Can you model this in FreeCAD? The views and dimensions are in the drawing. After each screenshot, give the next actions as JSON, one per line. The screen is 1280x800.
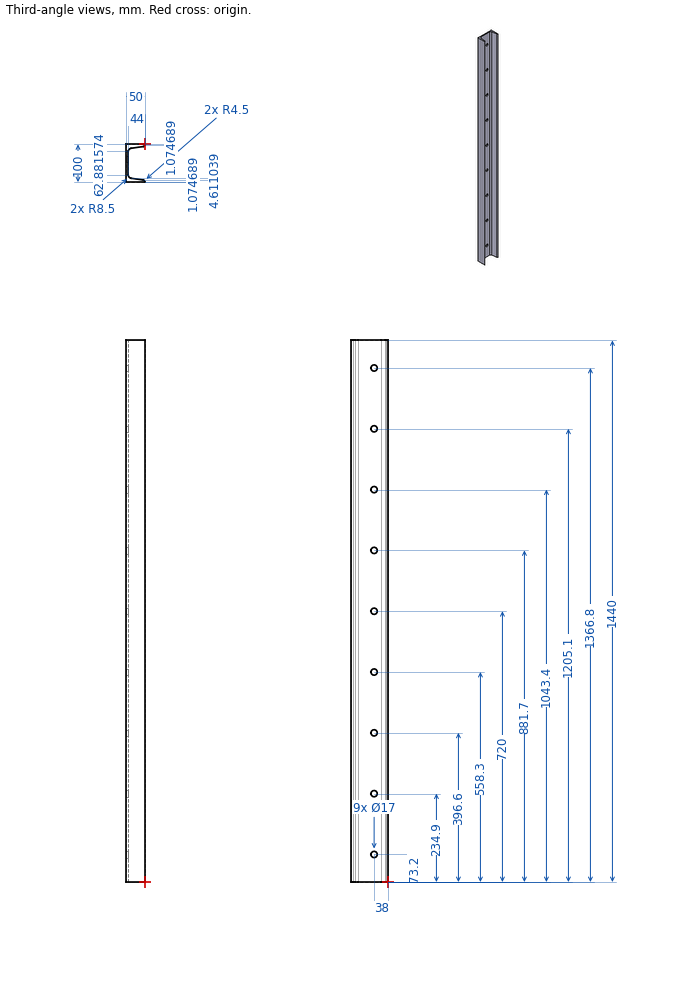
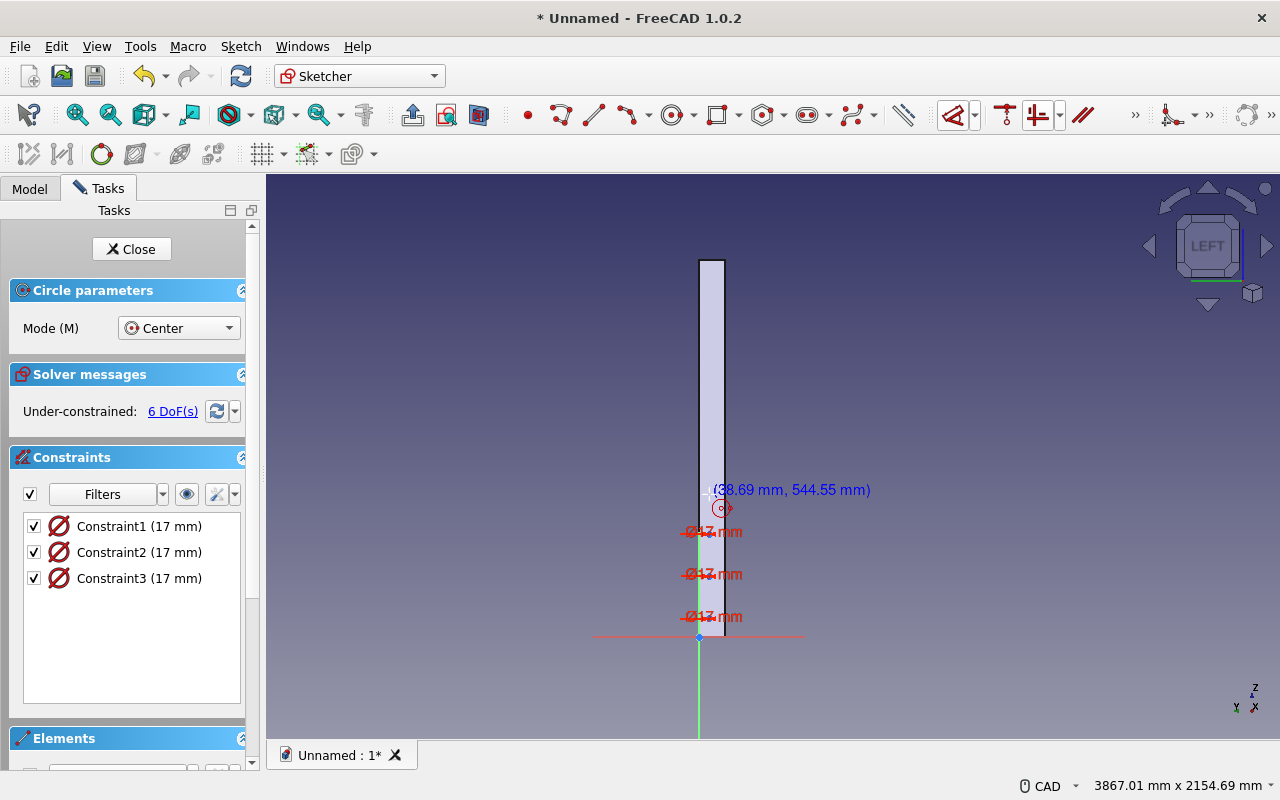
{"action": "scroll", "coordinate": [709, 491], "scroll_direction": "up", "scroll_amount": 3}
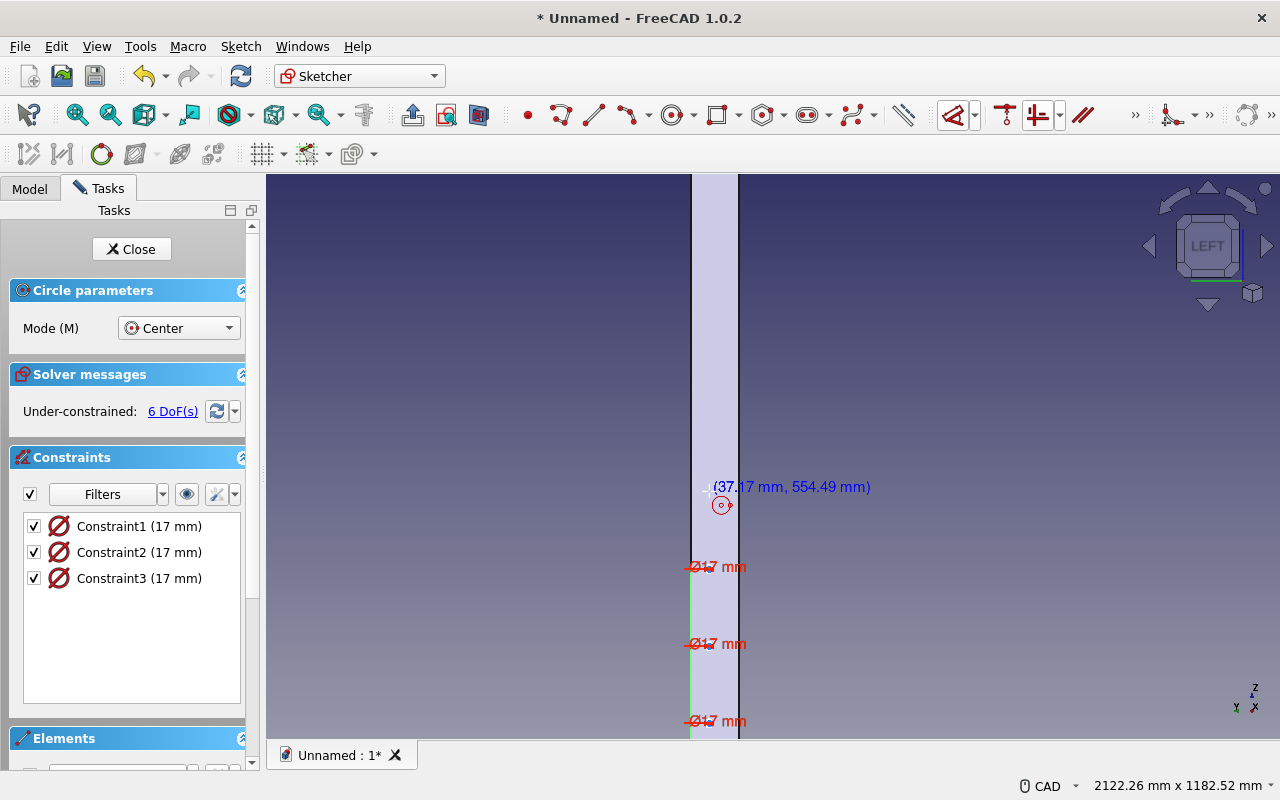
{"action": "left_click", "coordinate": [709, 491]}
{"action": "mouse_move", "coordinate": [712, 488]}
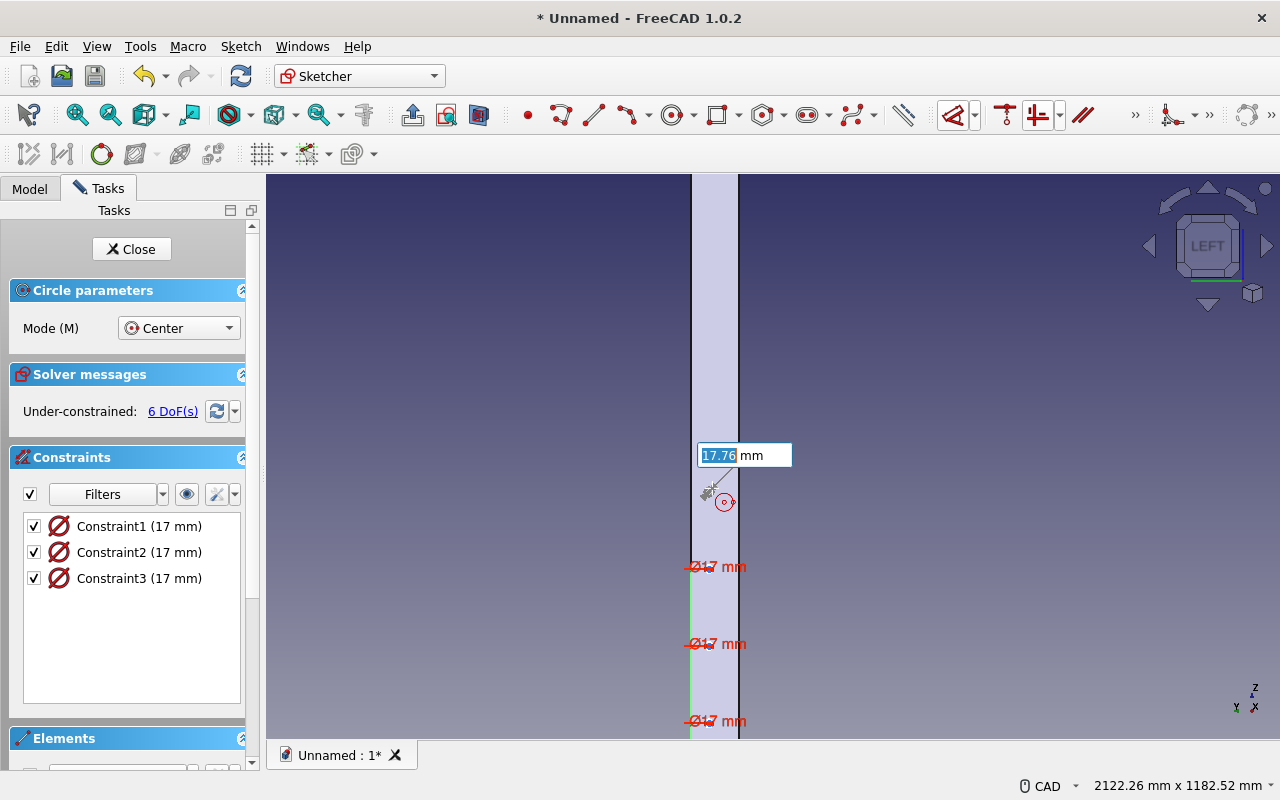
{"action": "type", "text": "17"}
{"action": "key", "text": "Return"}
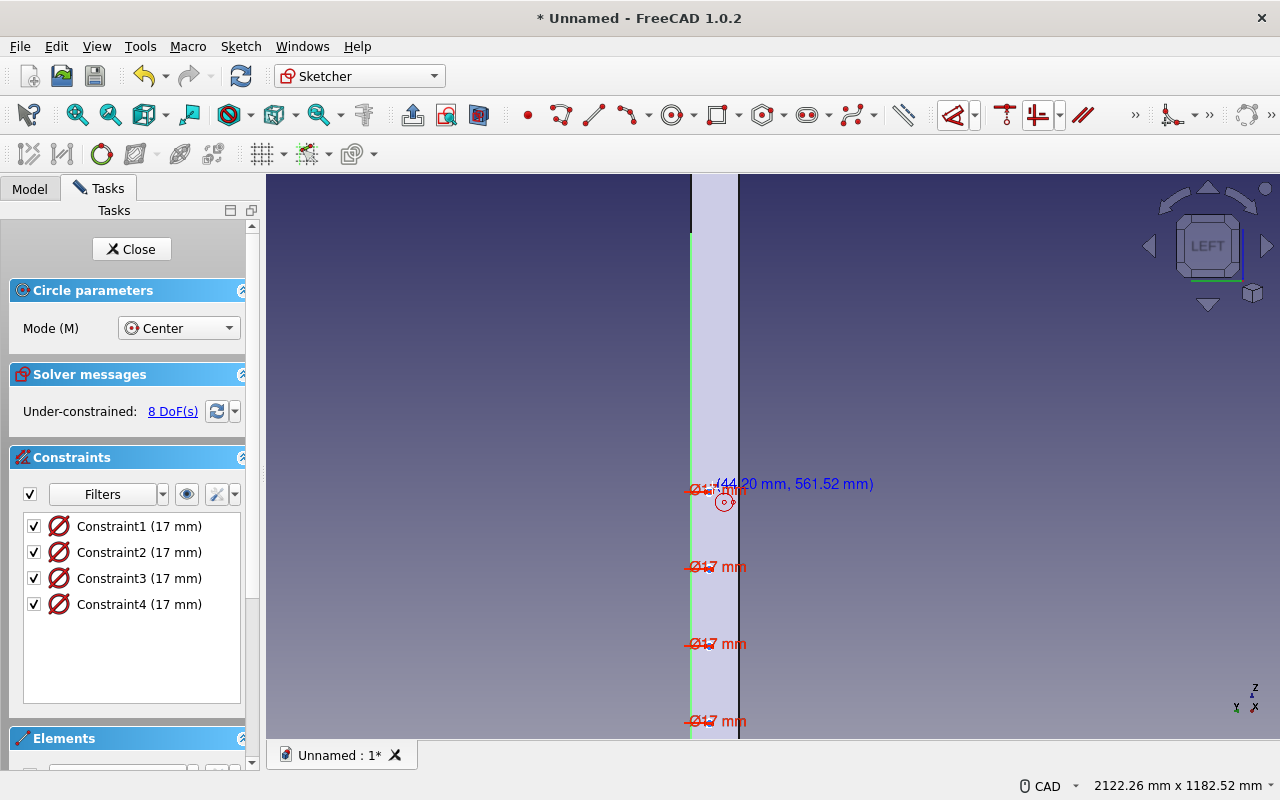
{"action": "scroll", "coordinate": [709, 413], "scroll_direction": "up", "scroll_amount": 9}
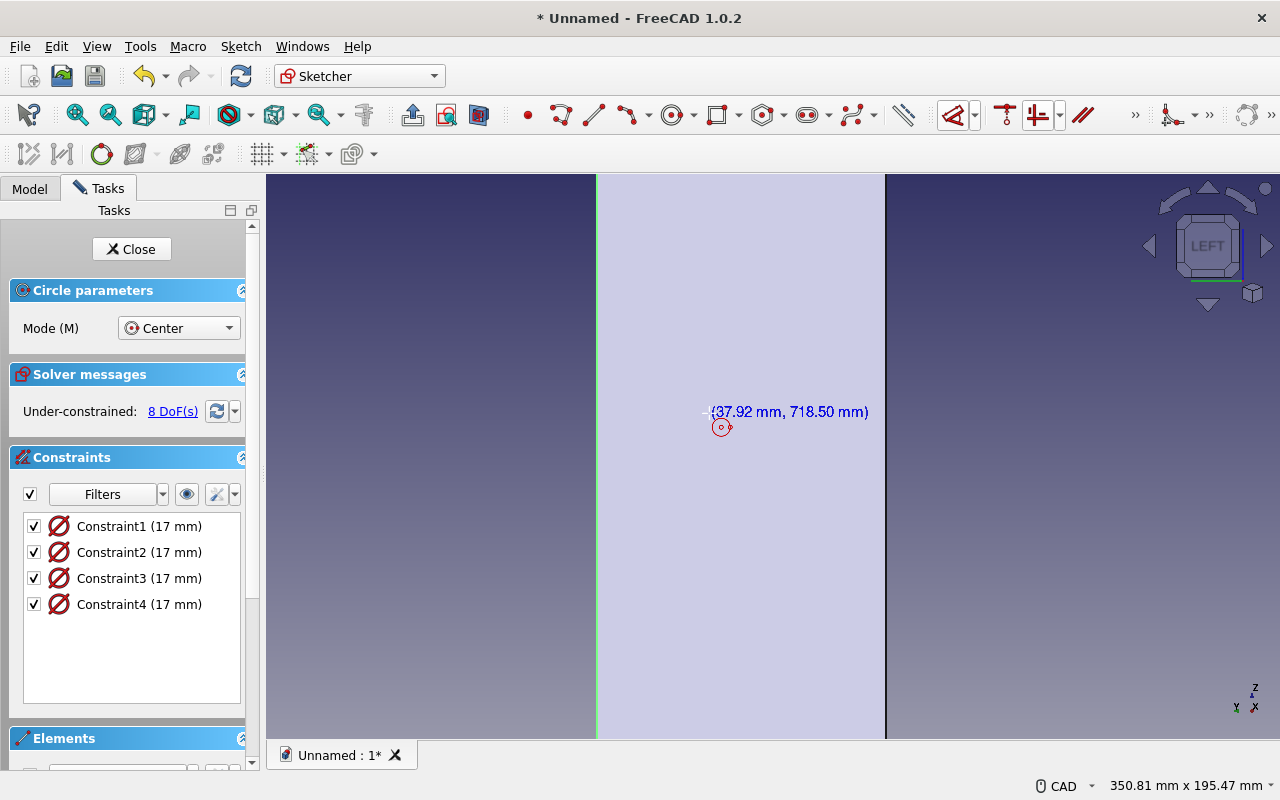
{"action": "scroll", "coordinate": [709, 452], "scroll_direction": "down", "scroll_amount": 12}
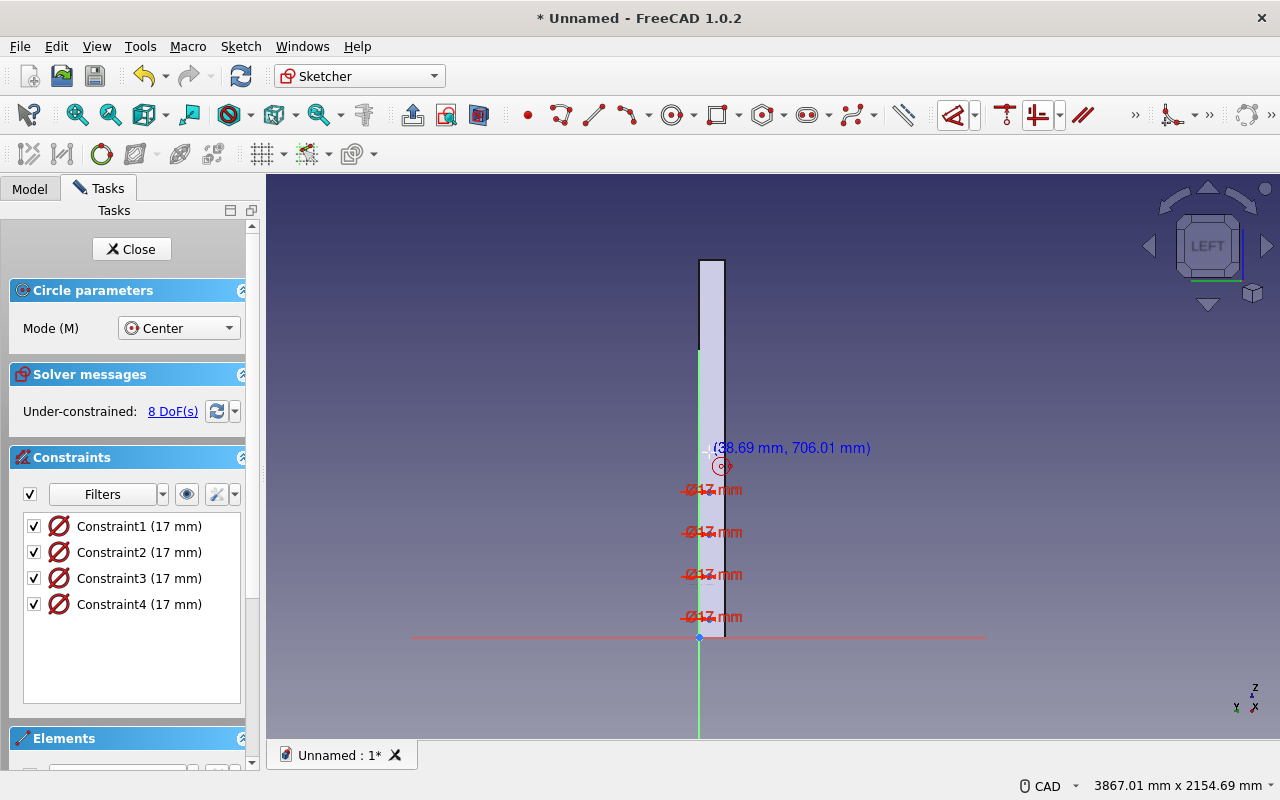
{"action": "scroll", "coordinate": [709, 449], "scroll_direction": "up", "scroll_amount": 3}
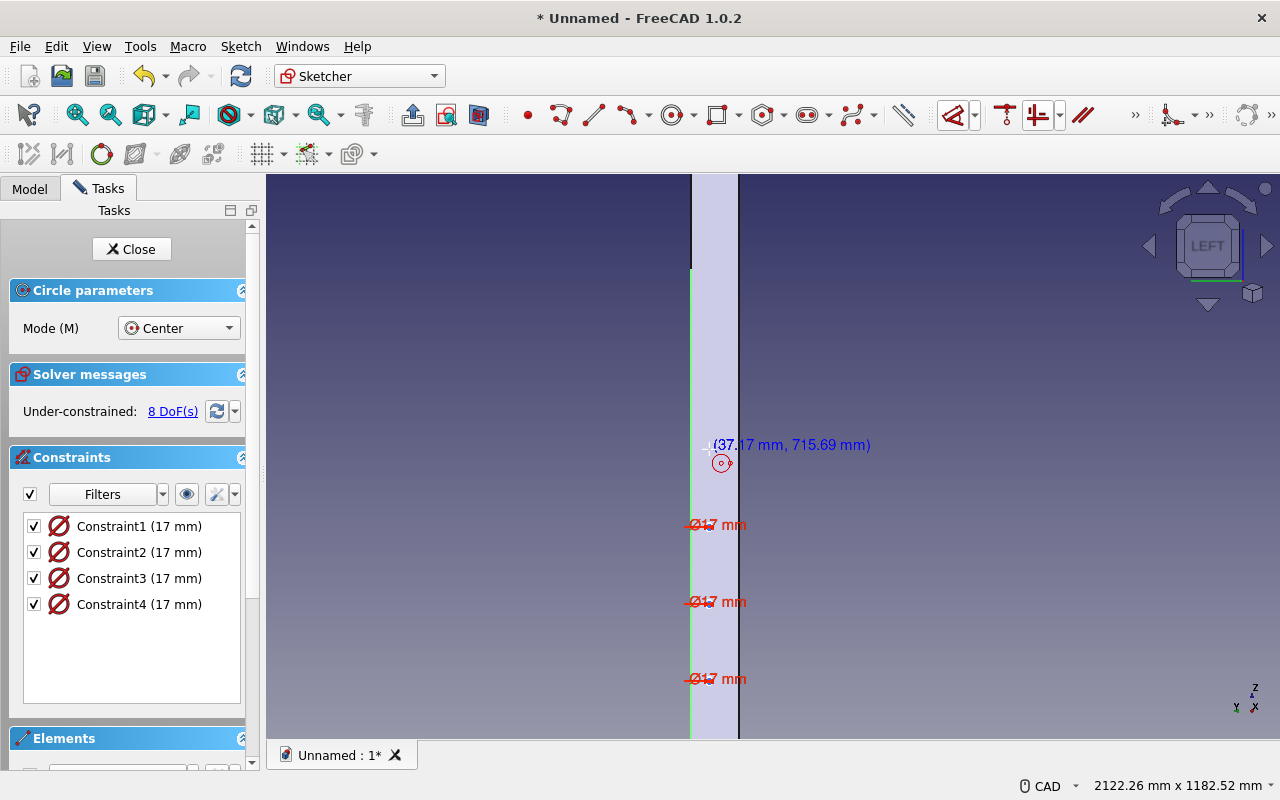
{"action": "left_click", "coordinate": [709, 448]}
{"action": "mouse_move", "coordinate": [712, 445]}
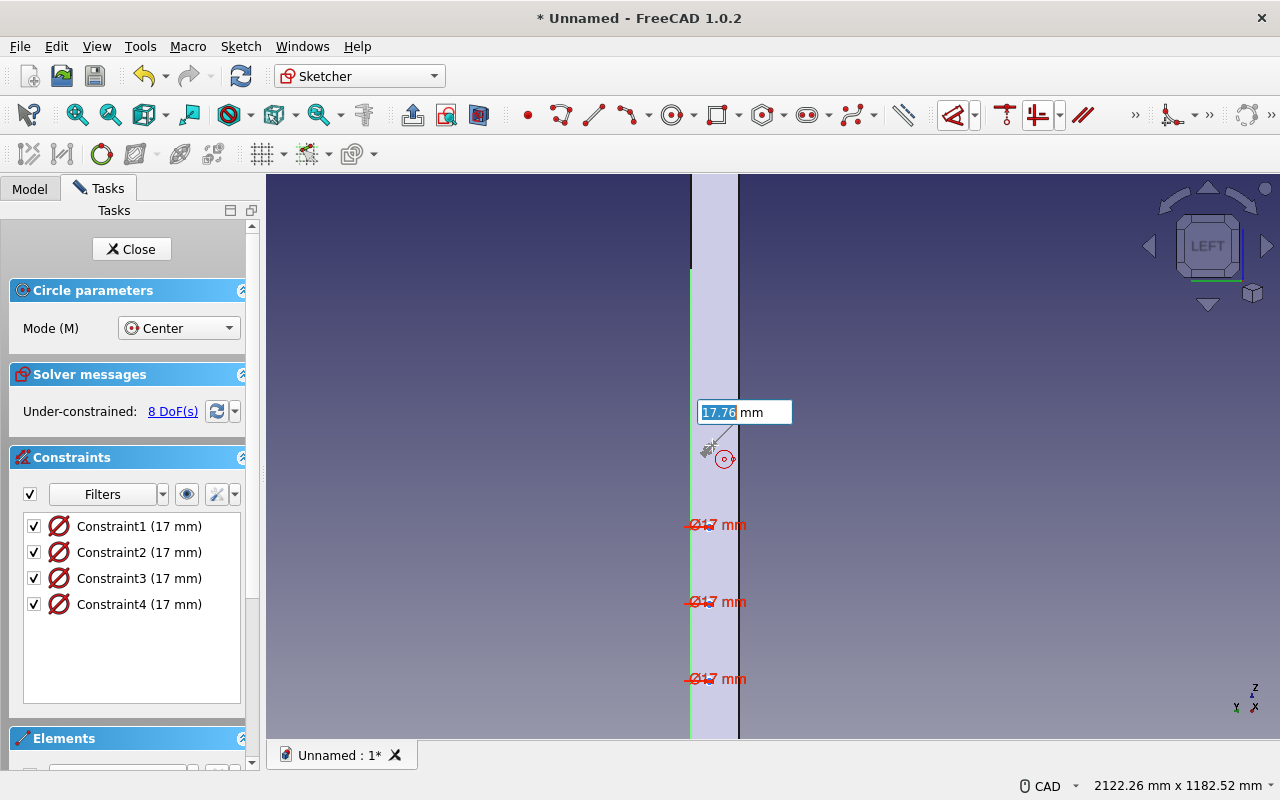
{"action": "type", "text": "17"}
{"action": "key", "text": "Return"}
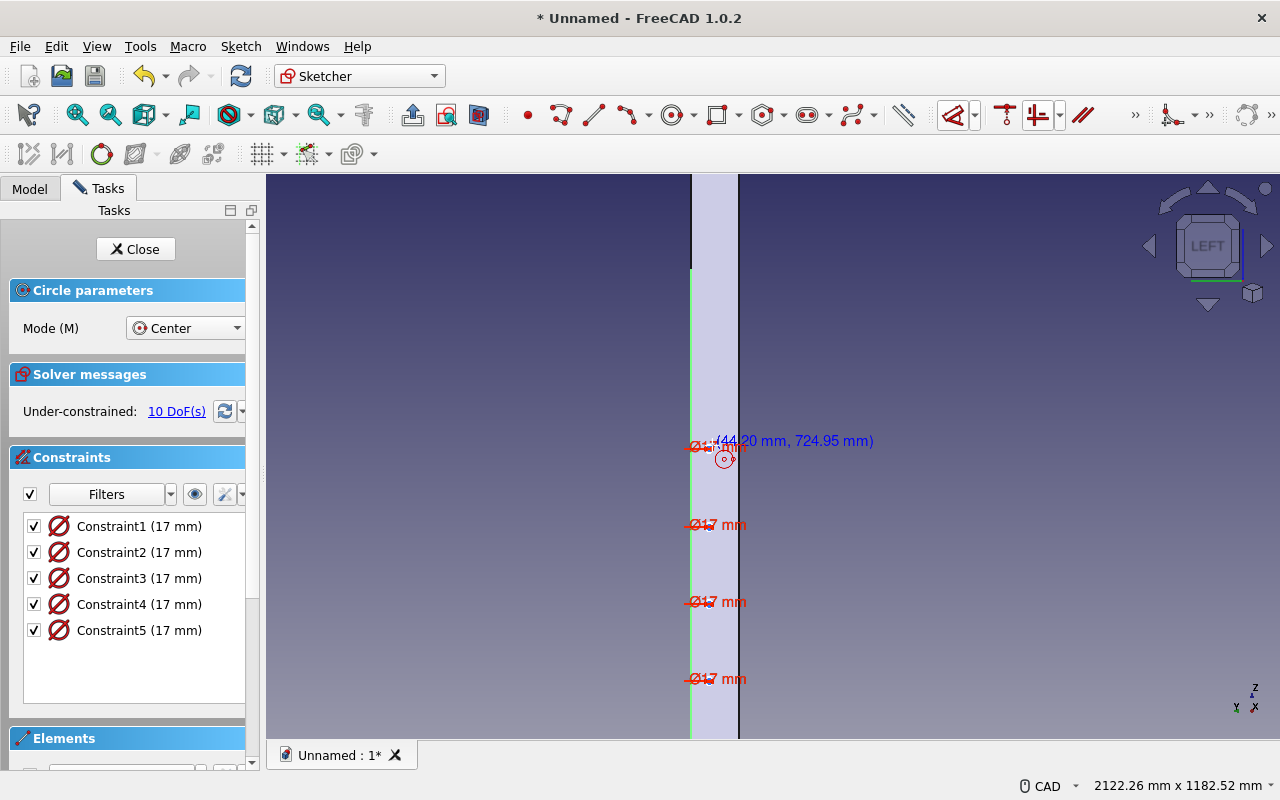
{"action": "scroll", "coordinate": [709, 371], "scroll_direction": "up", "scroll_amount": 9}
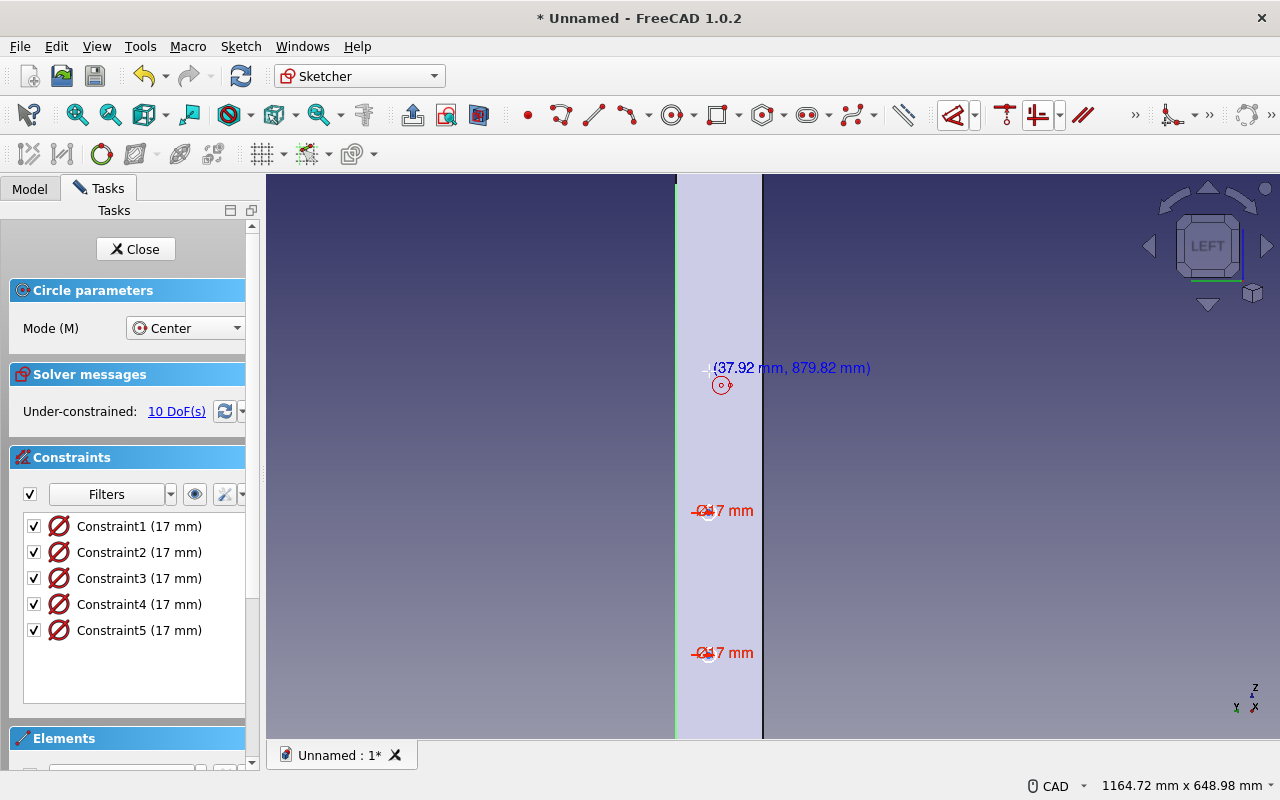
{"action": "scroll", "coordinate": [709, 409], "scroll_direction": "down", "scroll_amount": 12}